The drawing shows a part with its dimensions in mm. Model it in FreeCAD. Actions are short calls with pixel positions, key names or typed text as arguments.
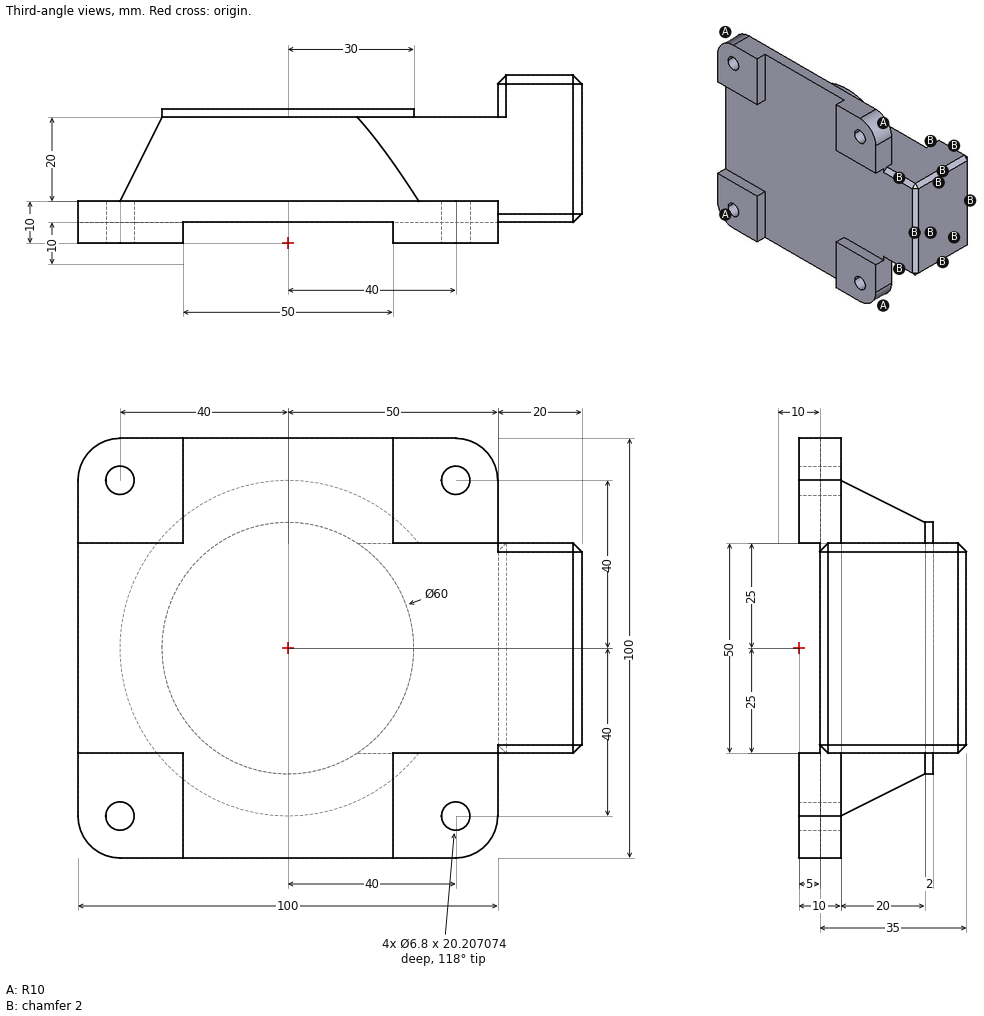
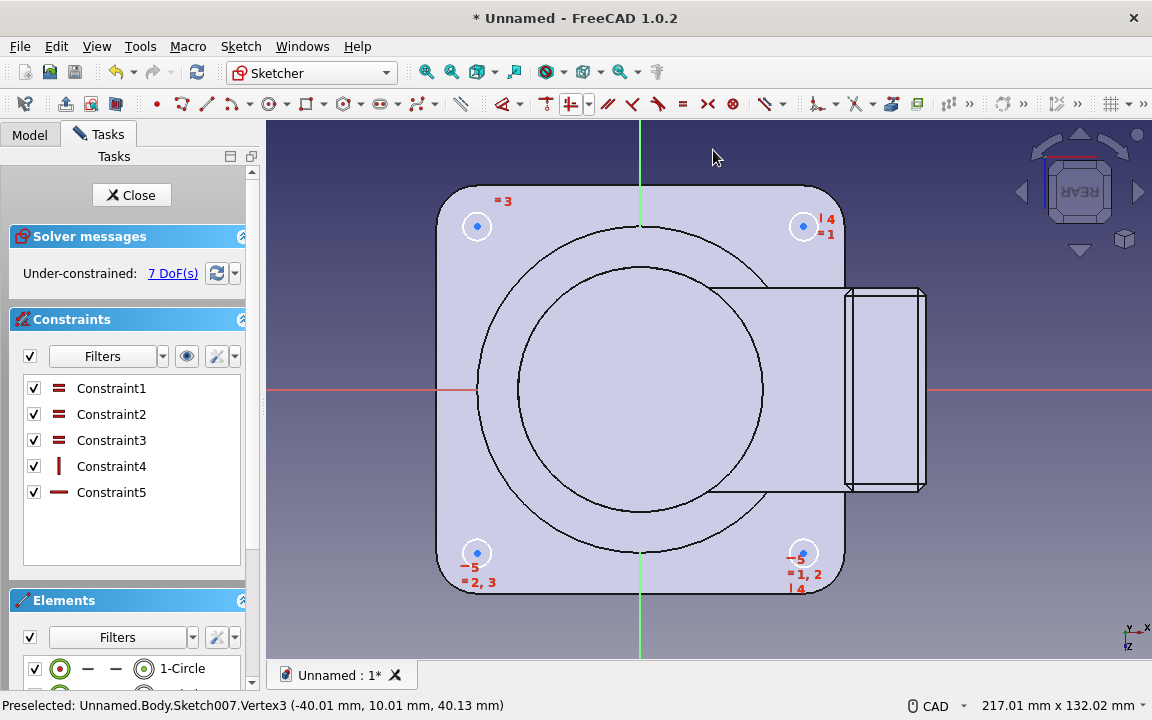
click(477, 553)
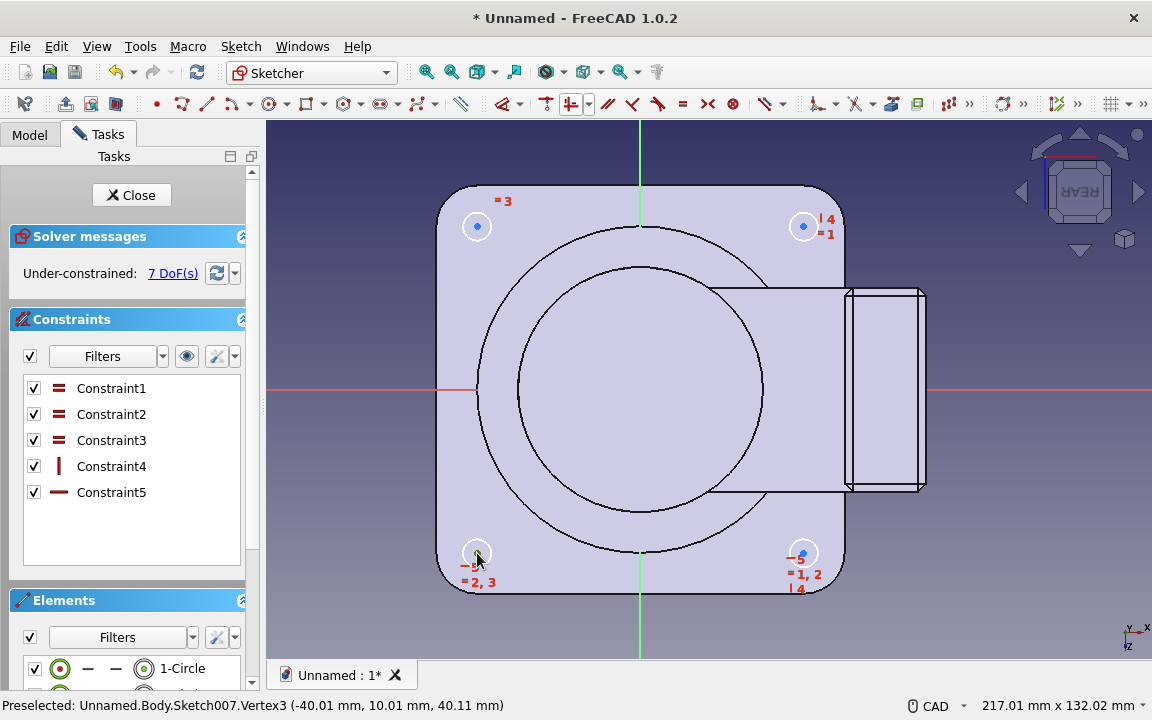
click(477, 227)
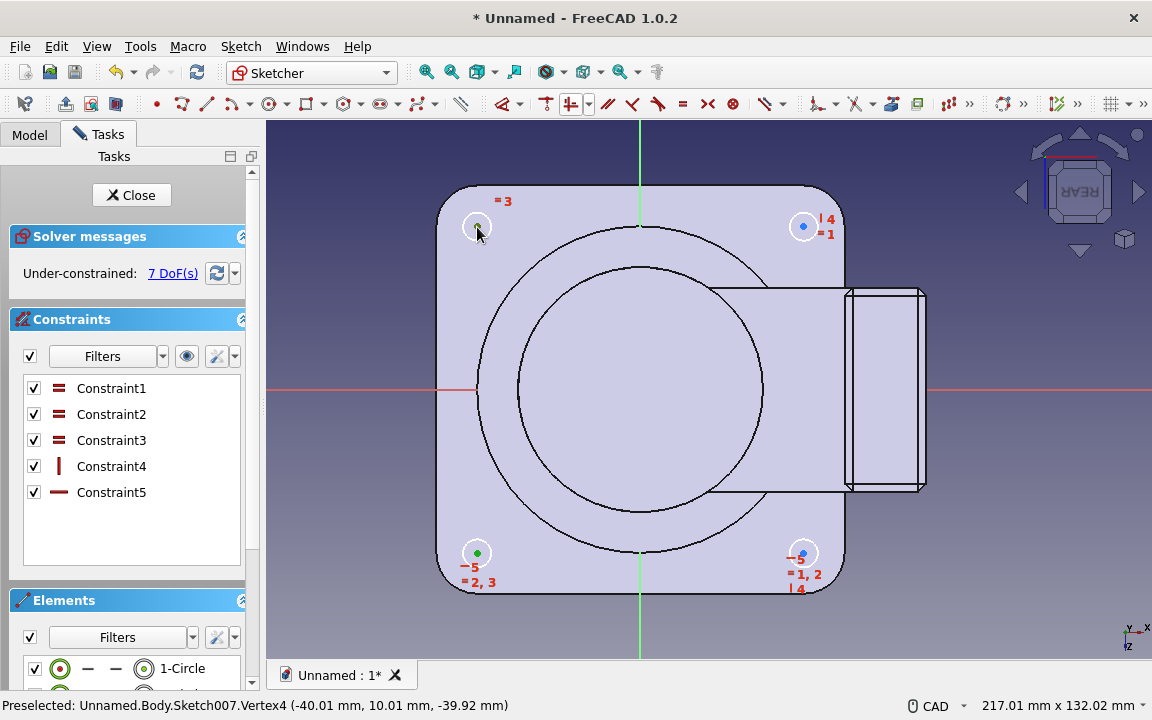
click(588, 104)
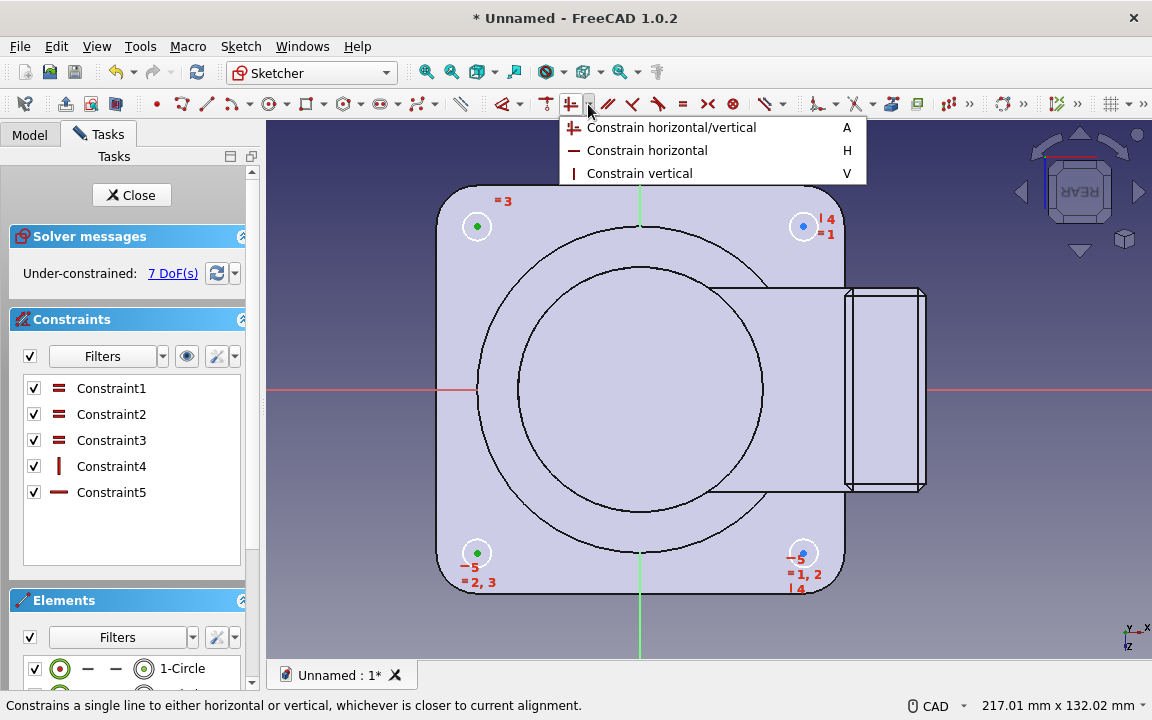
click(713, 174)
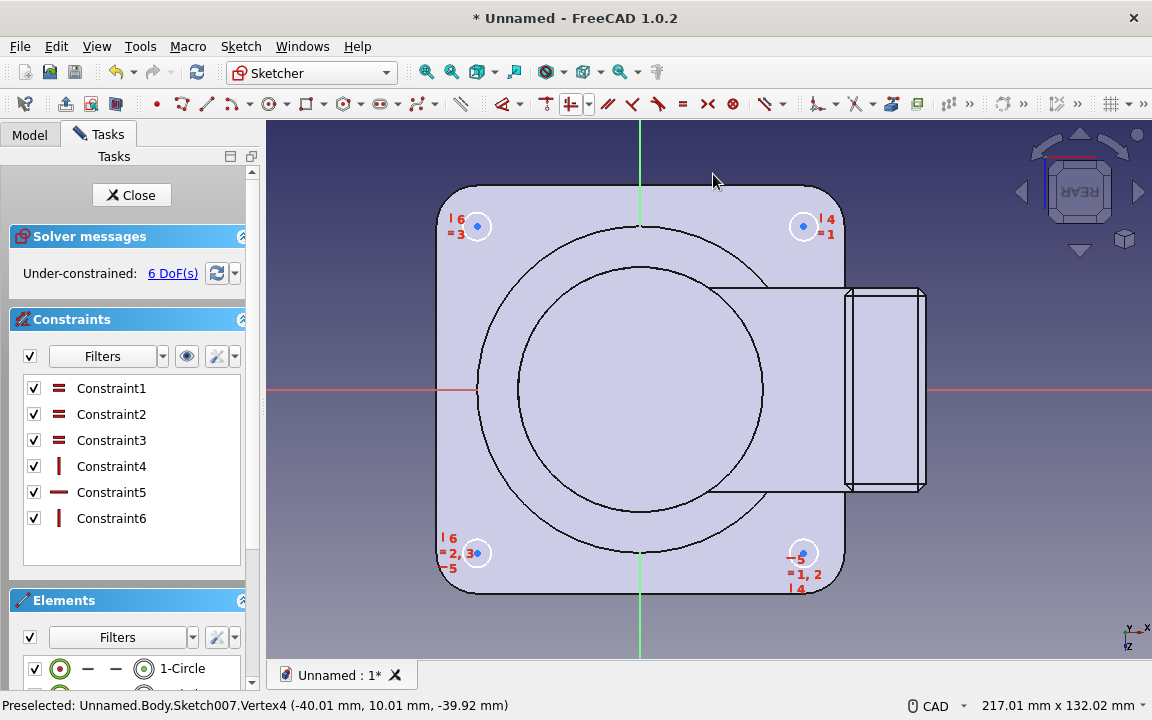
click(804, 227)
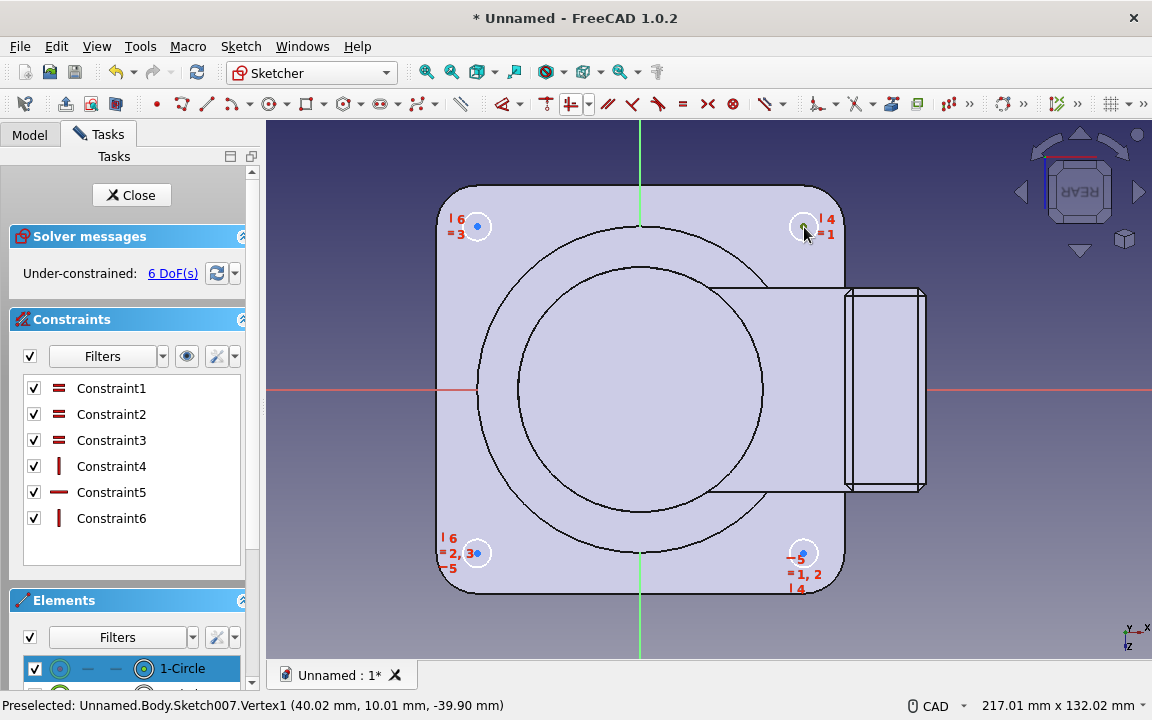
click(477, 227)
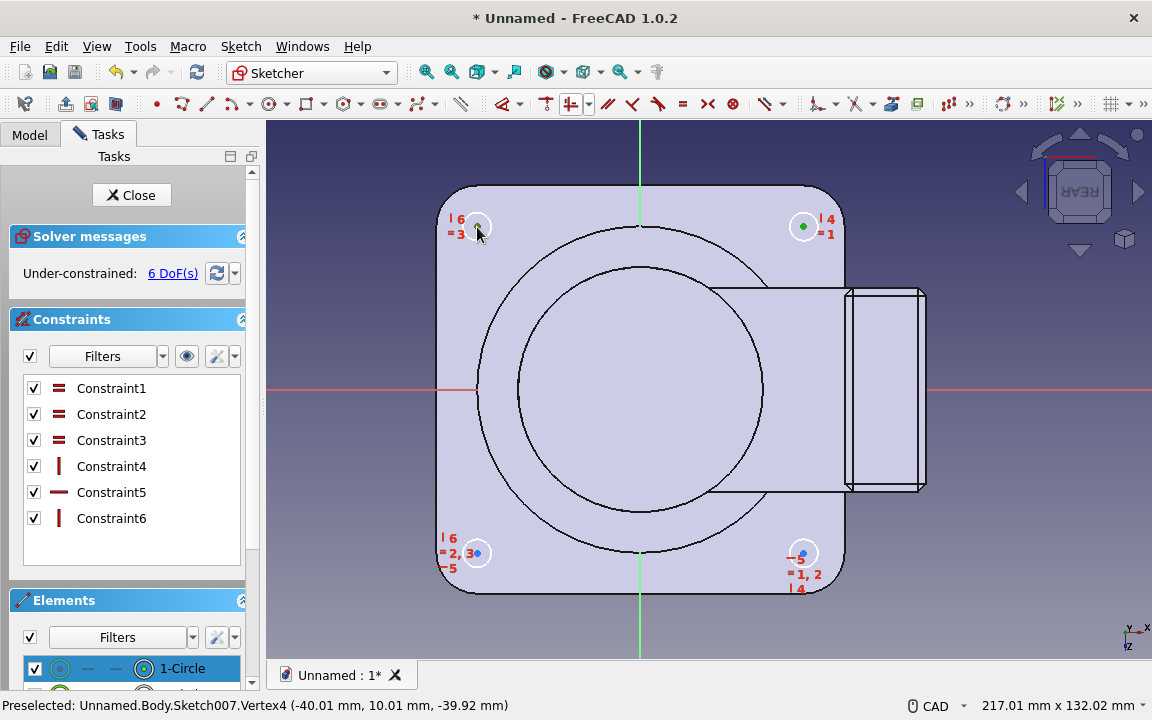
click(588, 104)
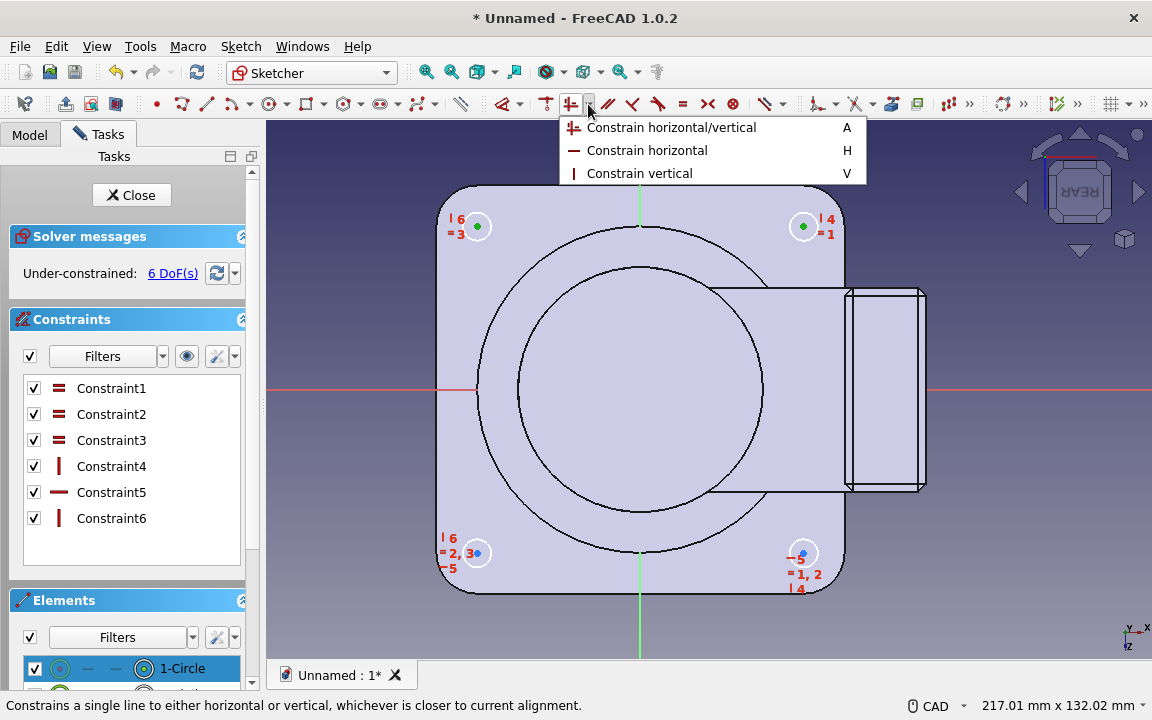
click(713, 150)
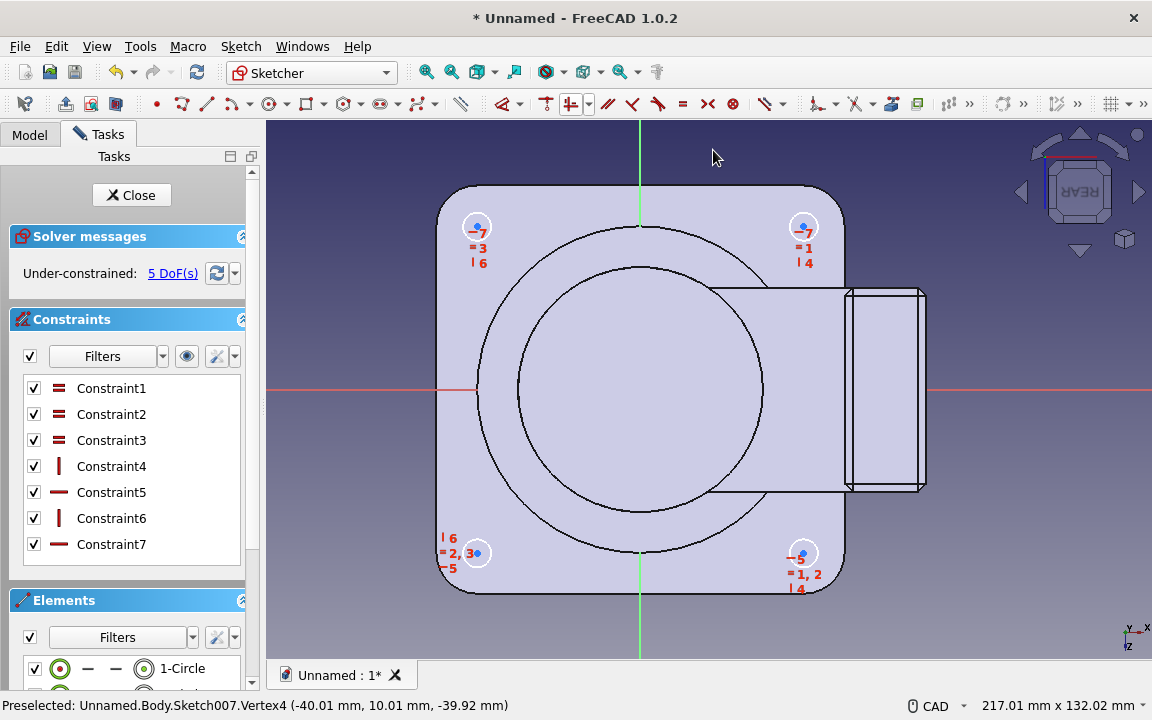
key(d)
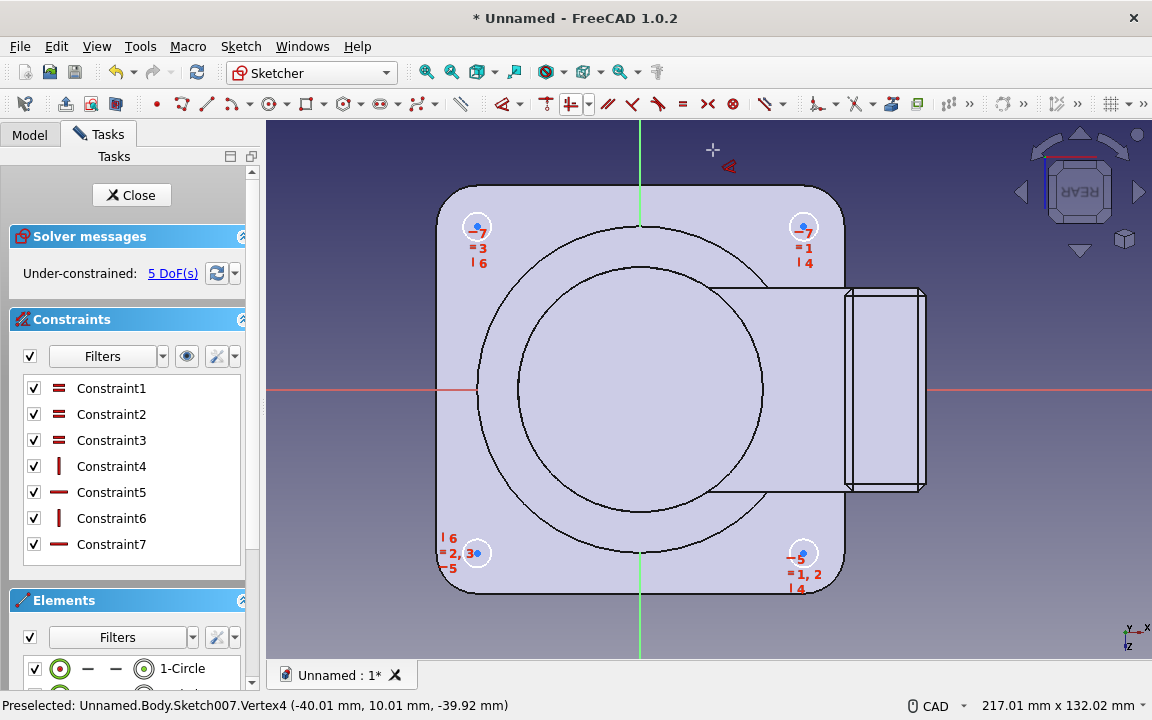
scroll(814, 217, up, 2)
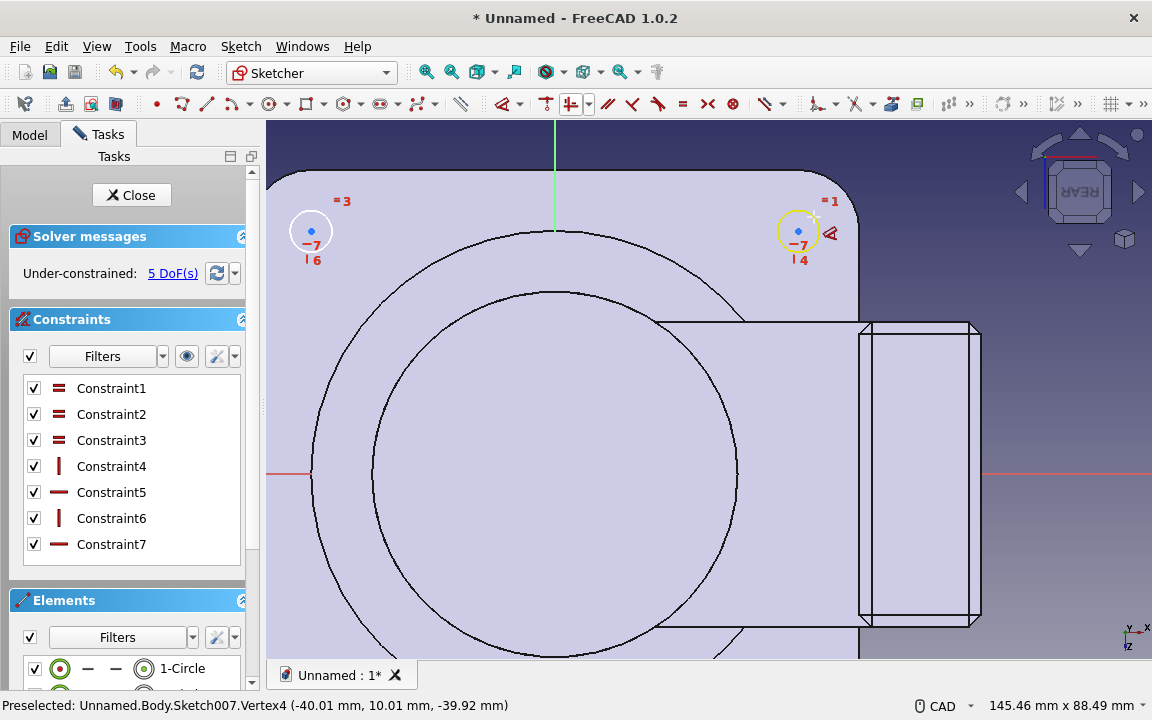
click(813, 217)
click(836, 194)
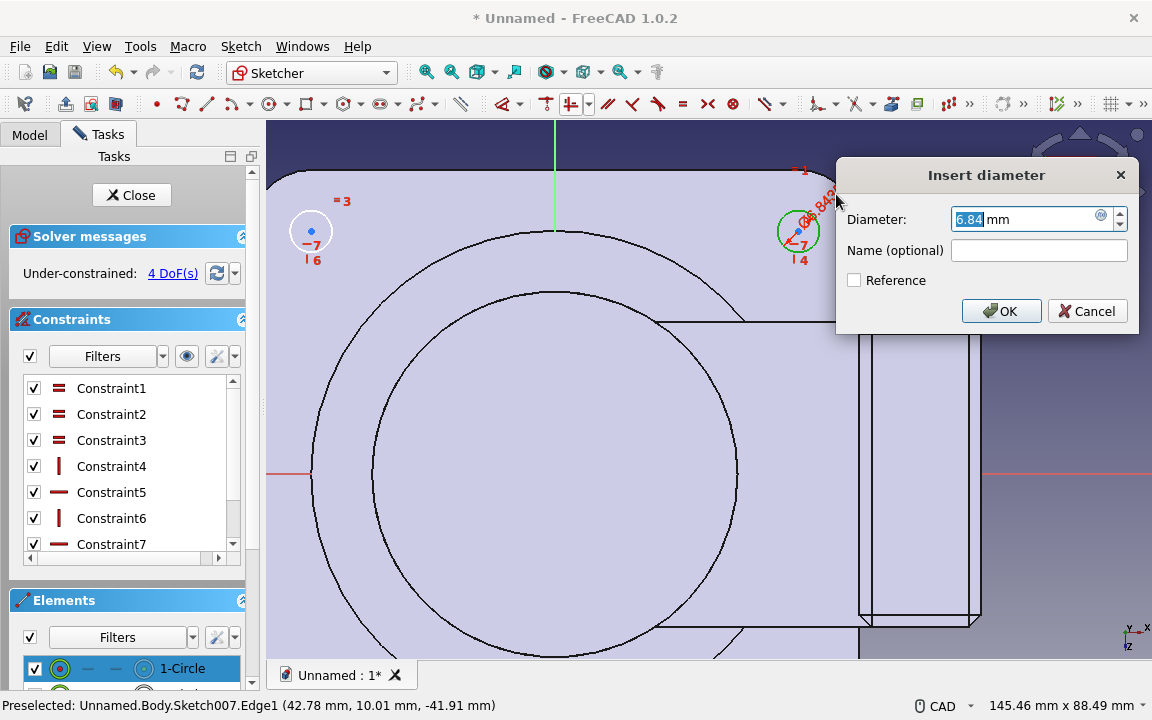
text(6.8)
key(Return)